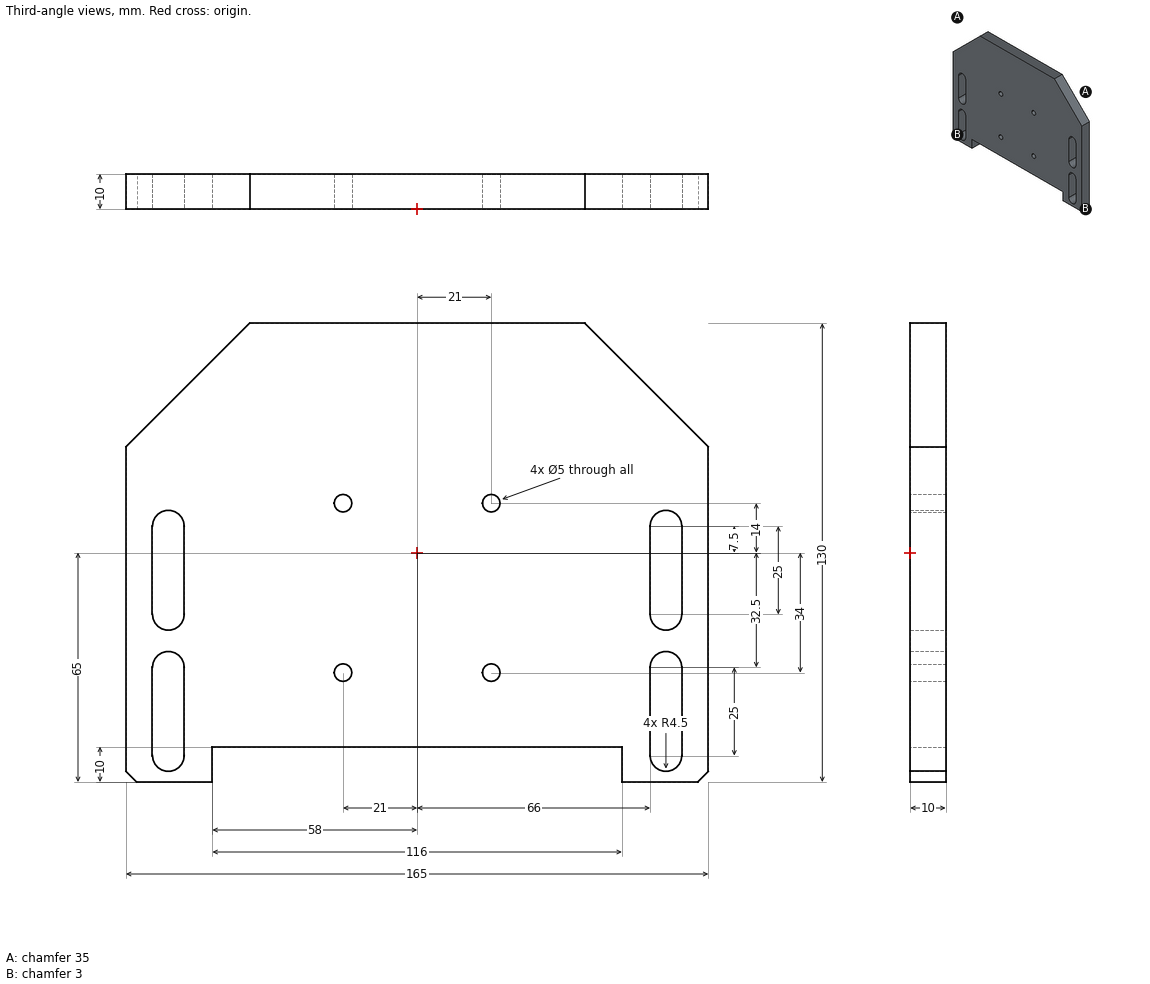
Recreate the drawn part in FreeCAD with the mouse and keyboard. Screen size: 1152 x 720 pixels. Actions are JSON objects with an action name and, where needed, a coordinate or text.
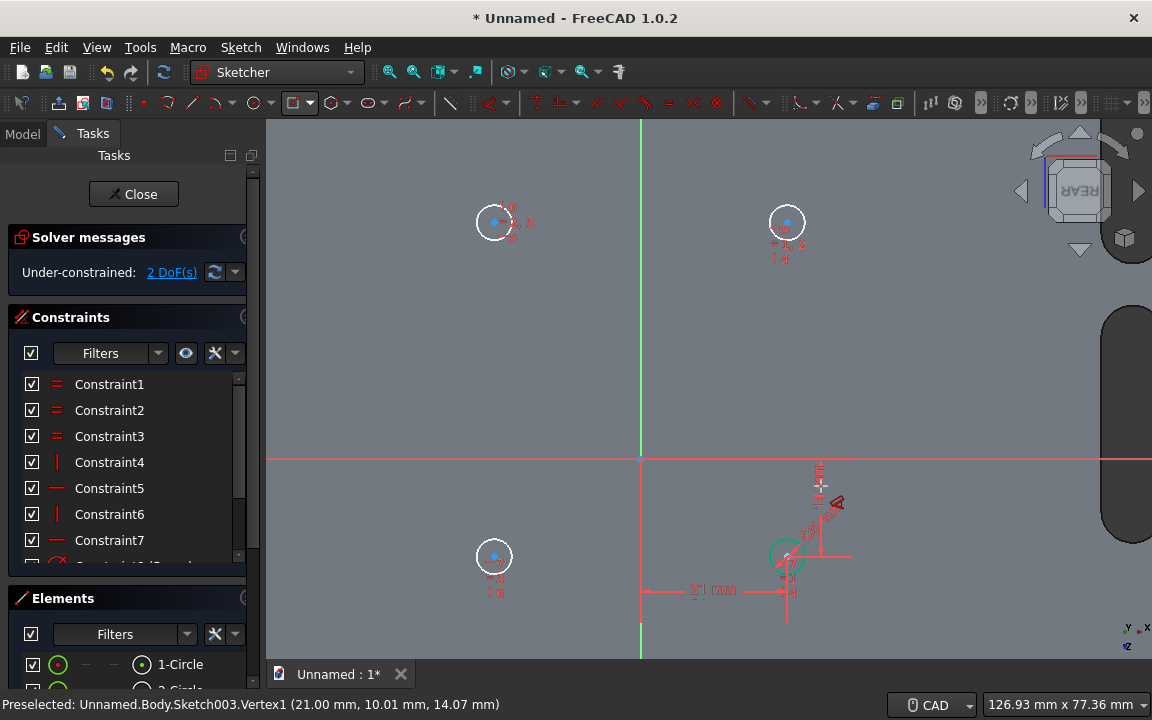
{"action": "left_click", "coordinate": [787, 223]}
{"action": "left_click", "coordinate": [821, 341]}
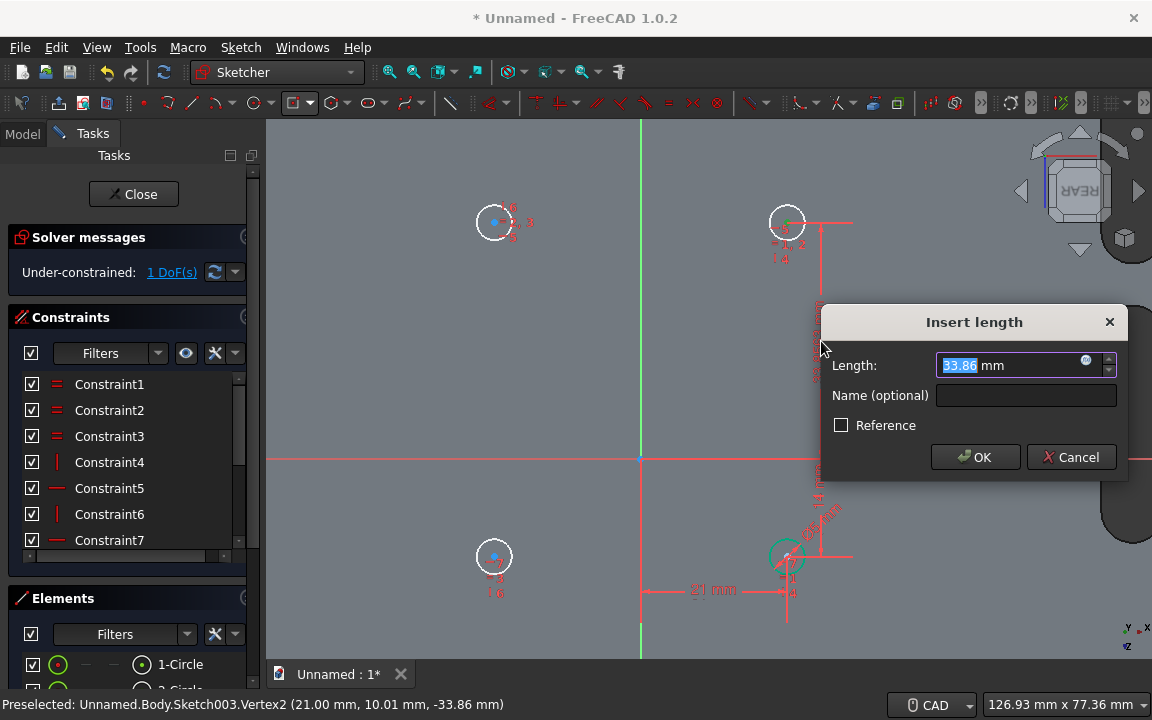
{"action": "type", "text": "34"}
{"action": "key", "text": "Return"}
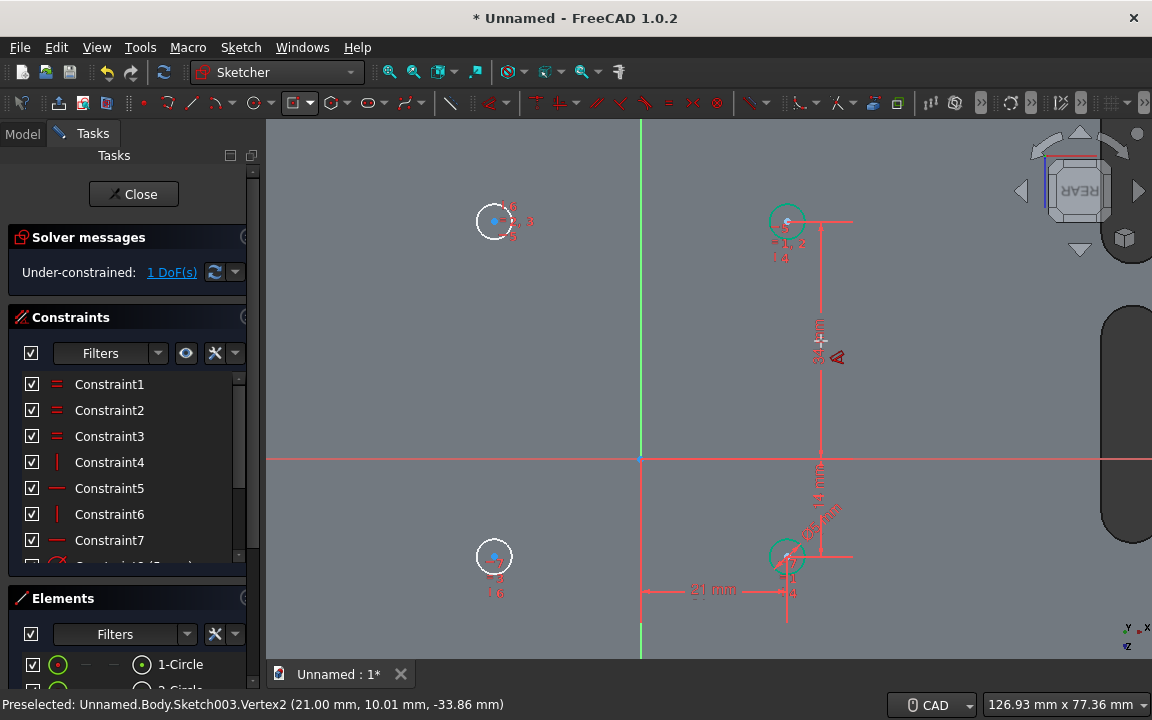
{"action": "left_click", "coordinate": [494, 222]}
{"action": "left_click", "coordinate": [567, 188]}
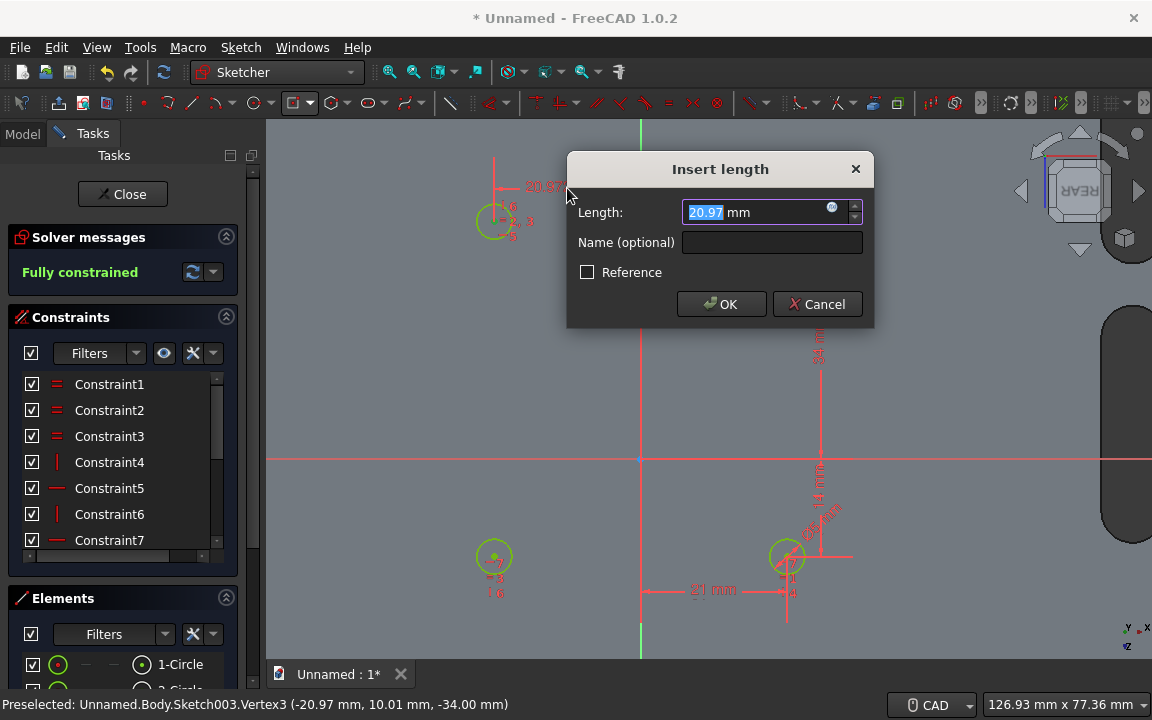
{"action": "type", "text": "21"}
{"action": "key", "text": "Return"}
{"action": "key", "text": "Escape"}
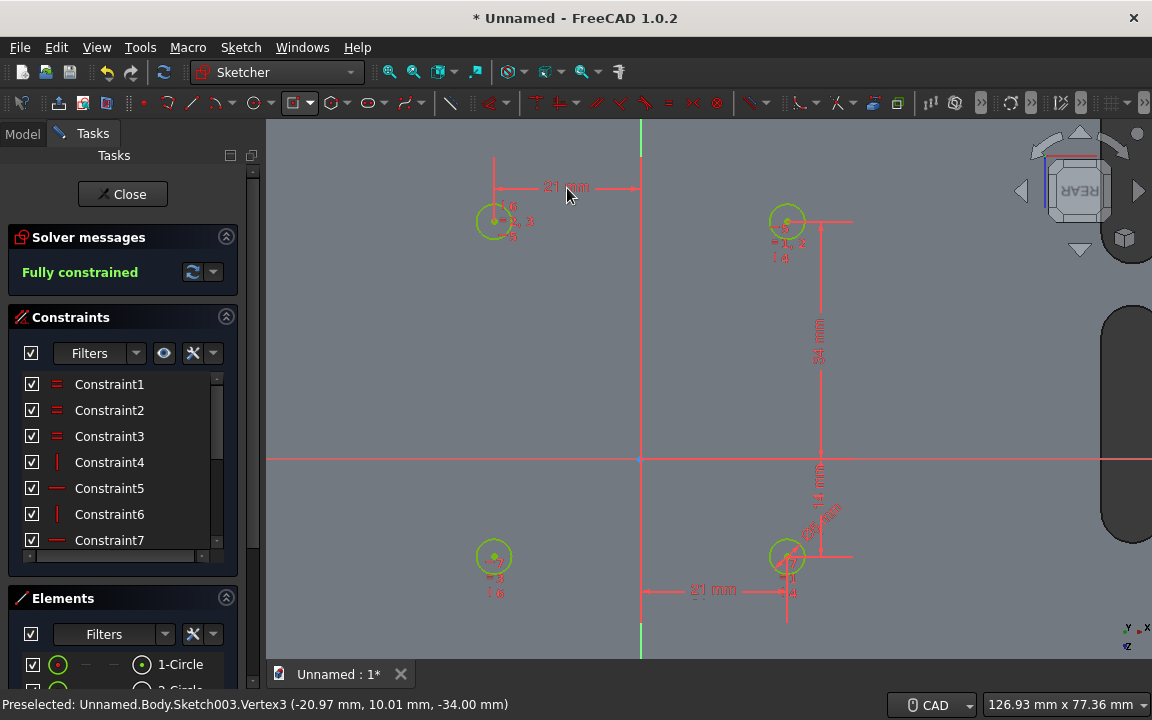
{"action": "left_click", "coordinate": [123, 194]}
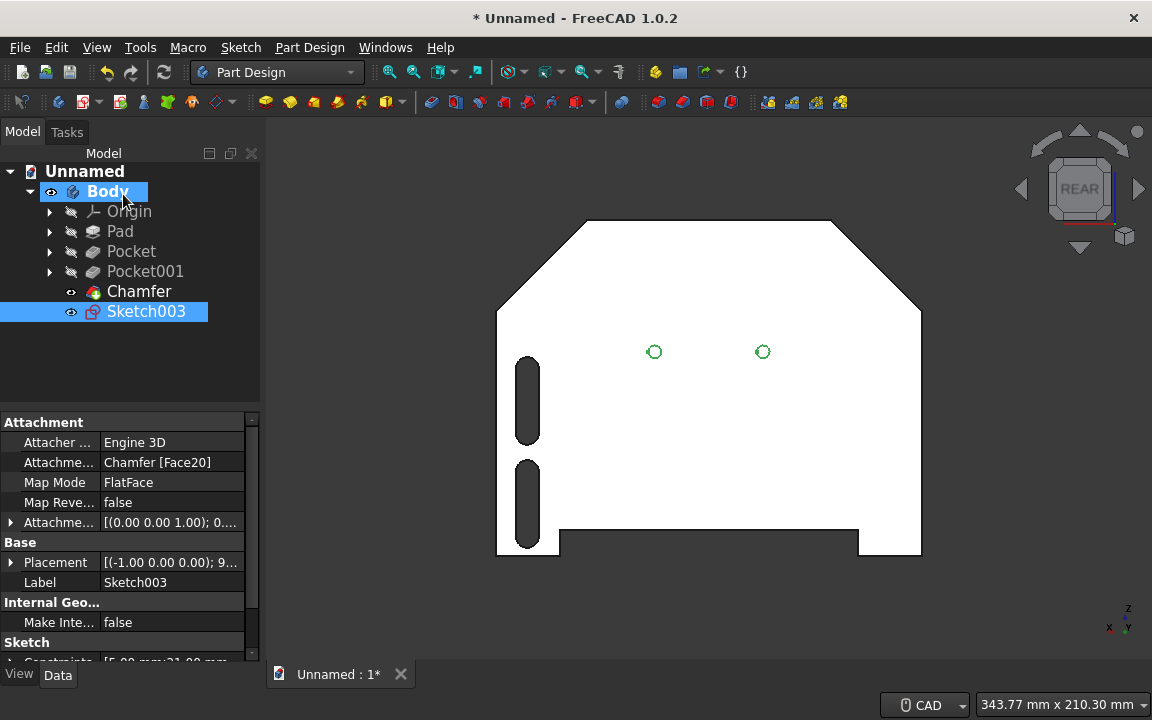
{"action": "left_click", "coordinate": [456, 102]}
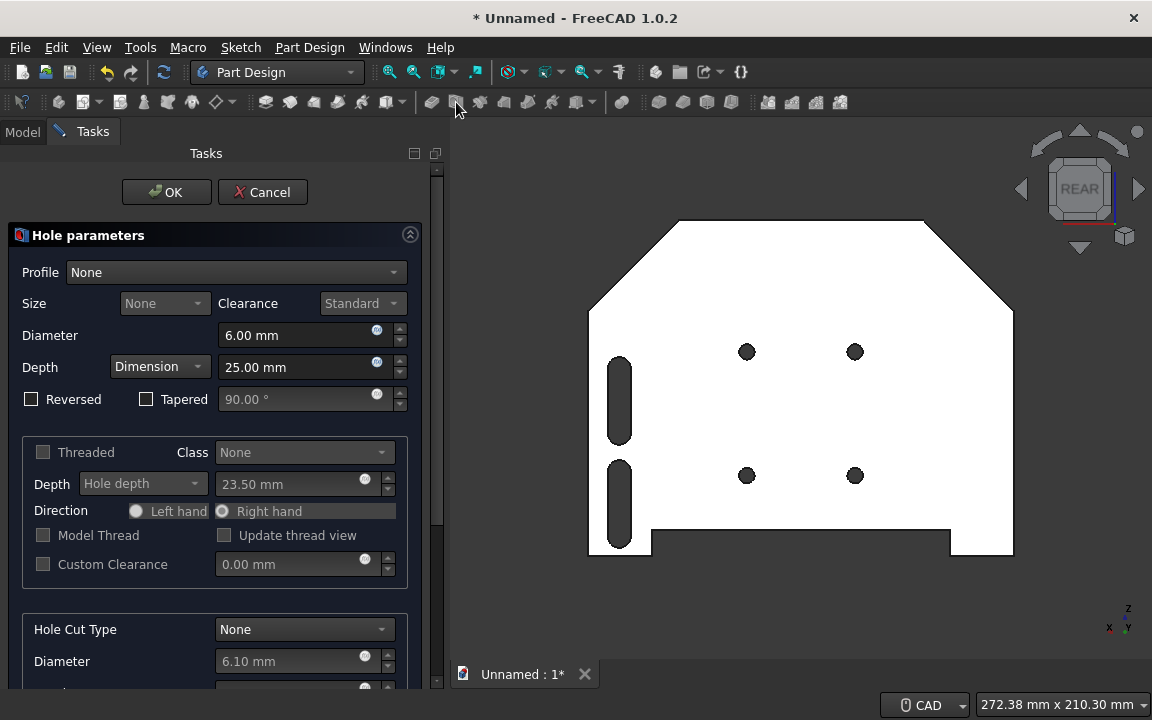
{"action": "triple_click", "coordinate": [305, 335]}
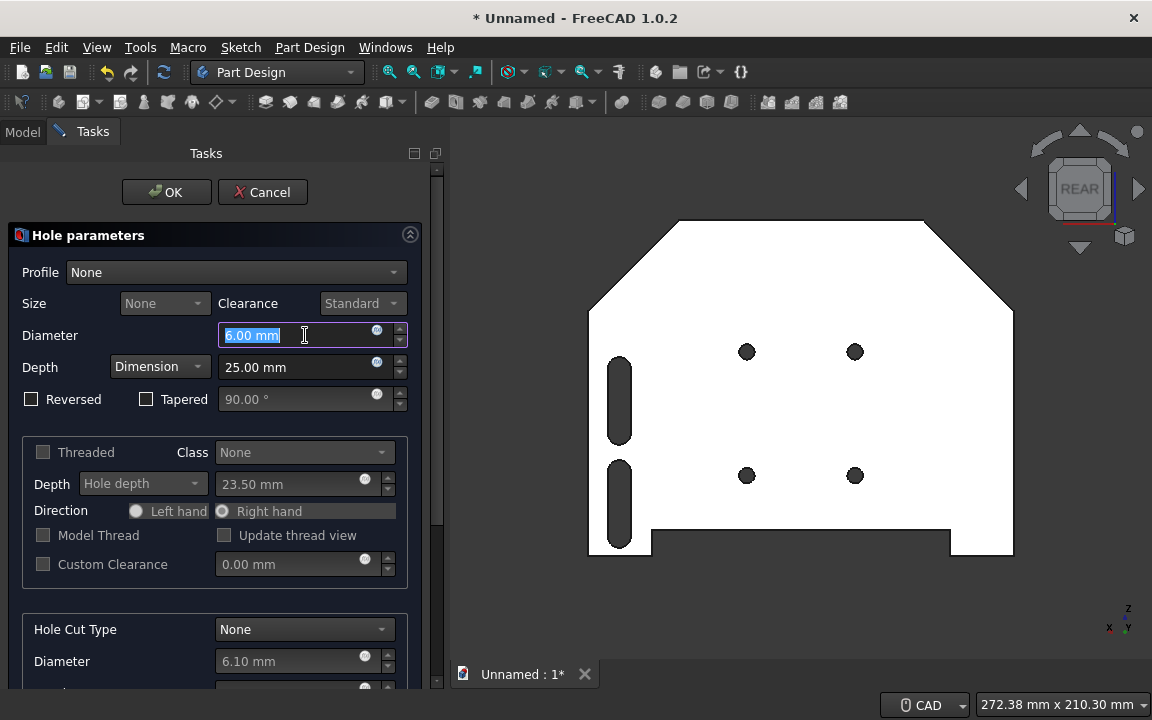
{"action": "type", "text": "5"}
{"action": "key", "text": "Tab"}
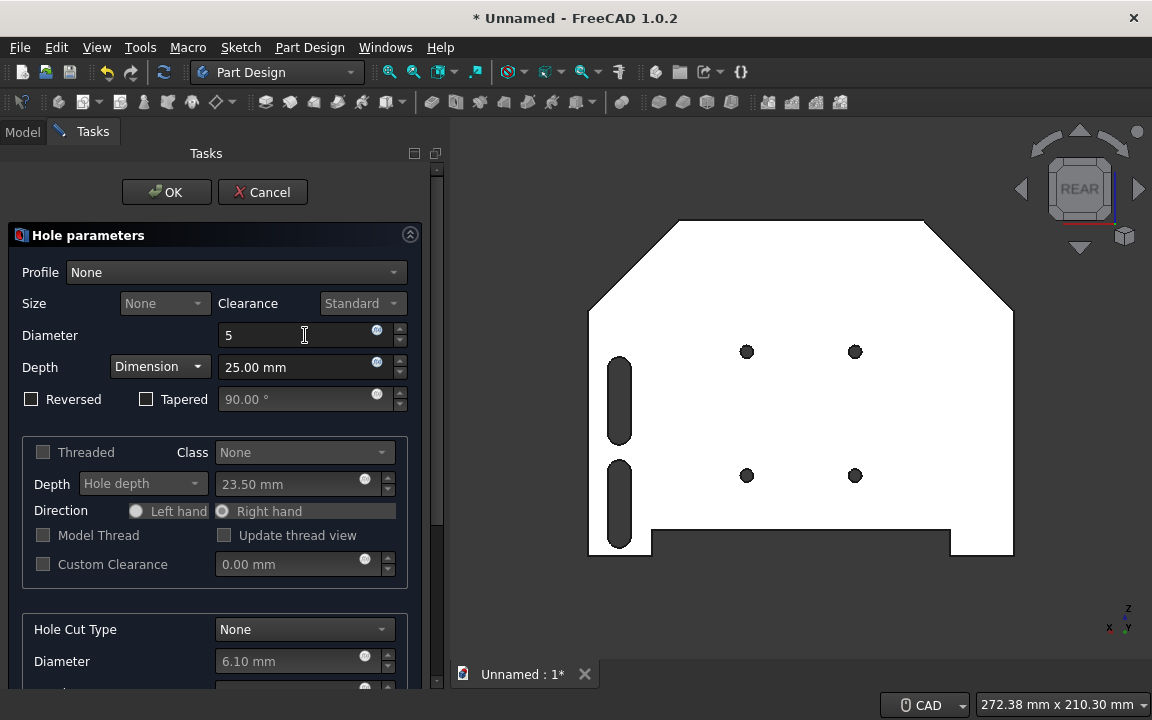
{"action": "left_click", "coordinate": [161, 366]}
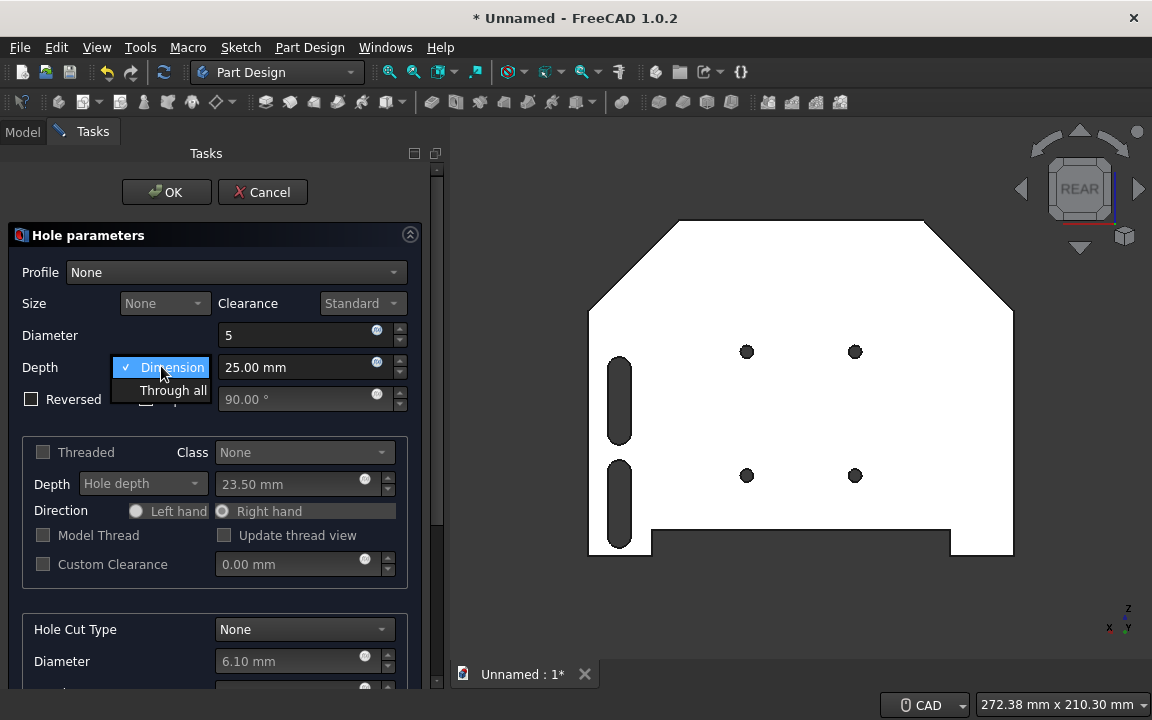
{"action": "left_click", "coordinate": [160, 390]}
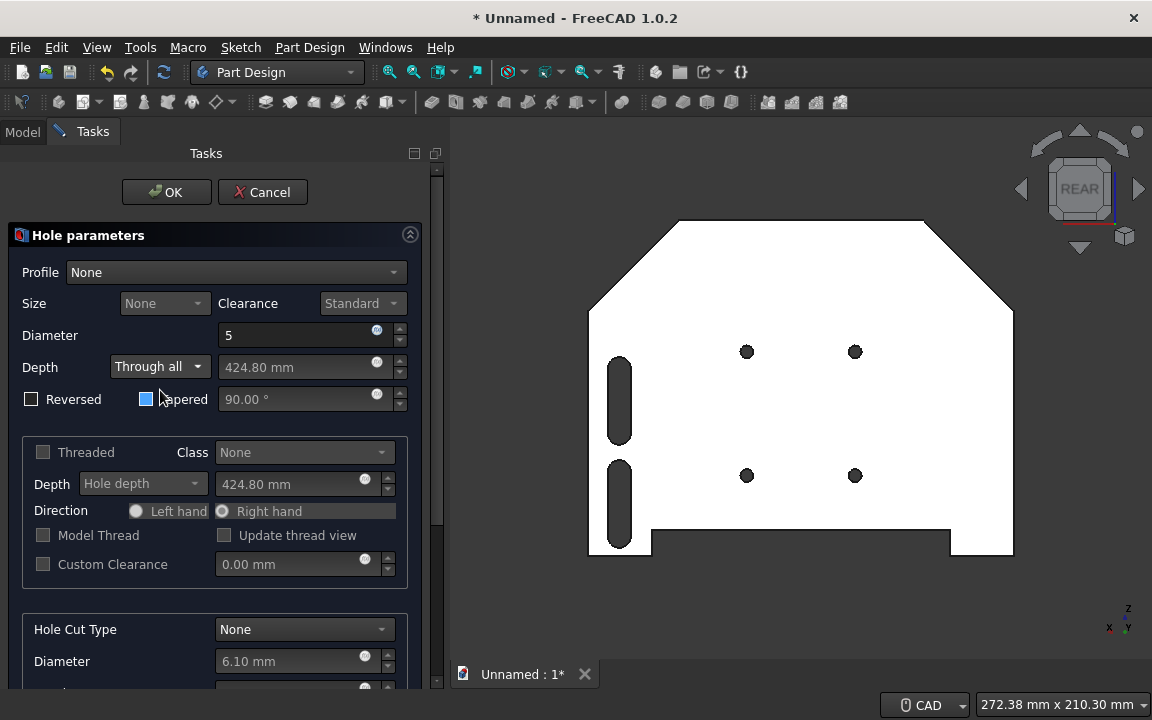
{"action": "left_click", "coordinate": [167, 192]}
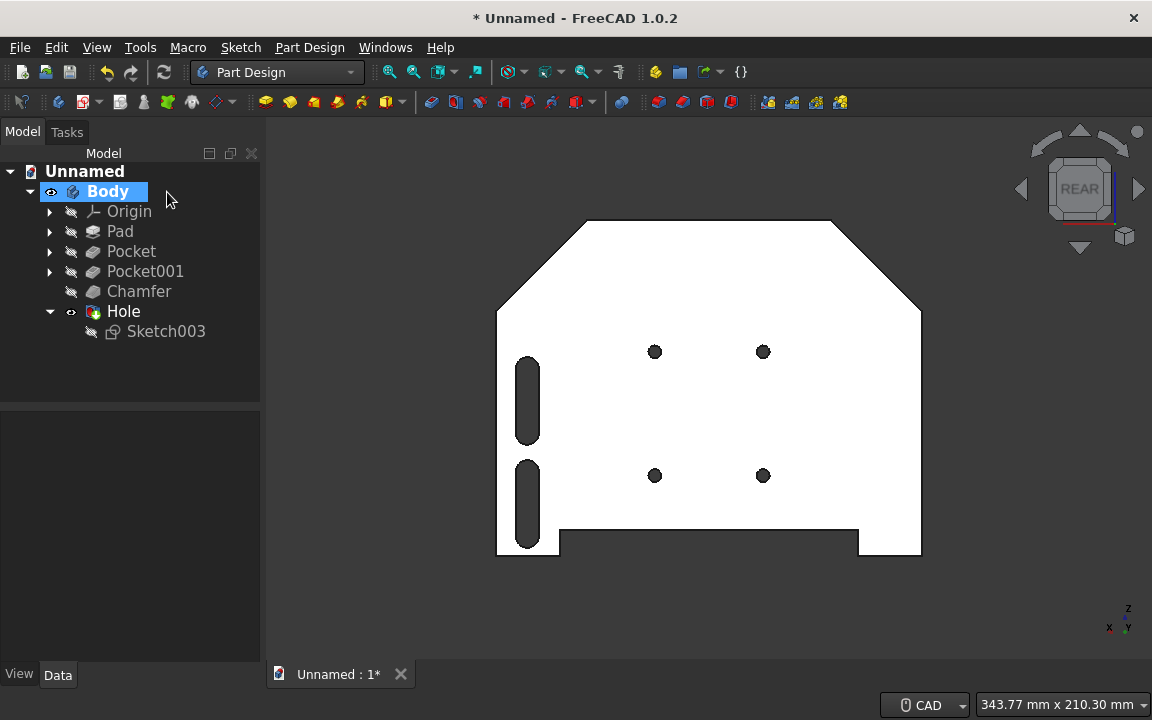
{"action": "key", "text": "0"}